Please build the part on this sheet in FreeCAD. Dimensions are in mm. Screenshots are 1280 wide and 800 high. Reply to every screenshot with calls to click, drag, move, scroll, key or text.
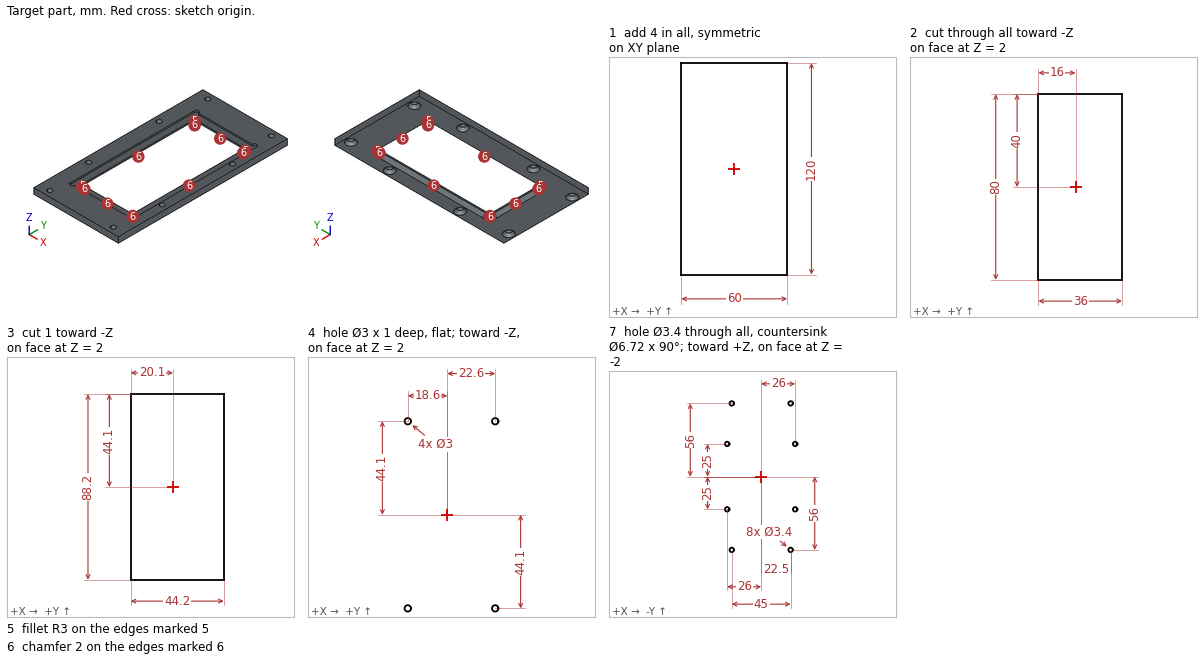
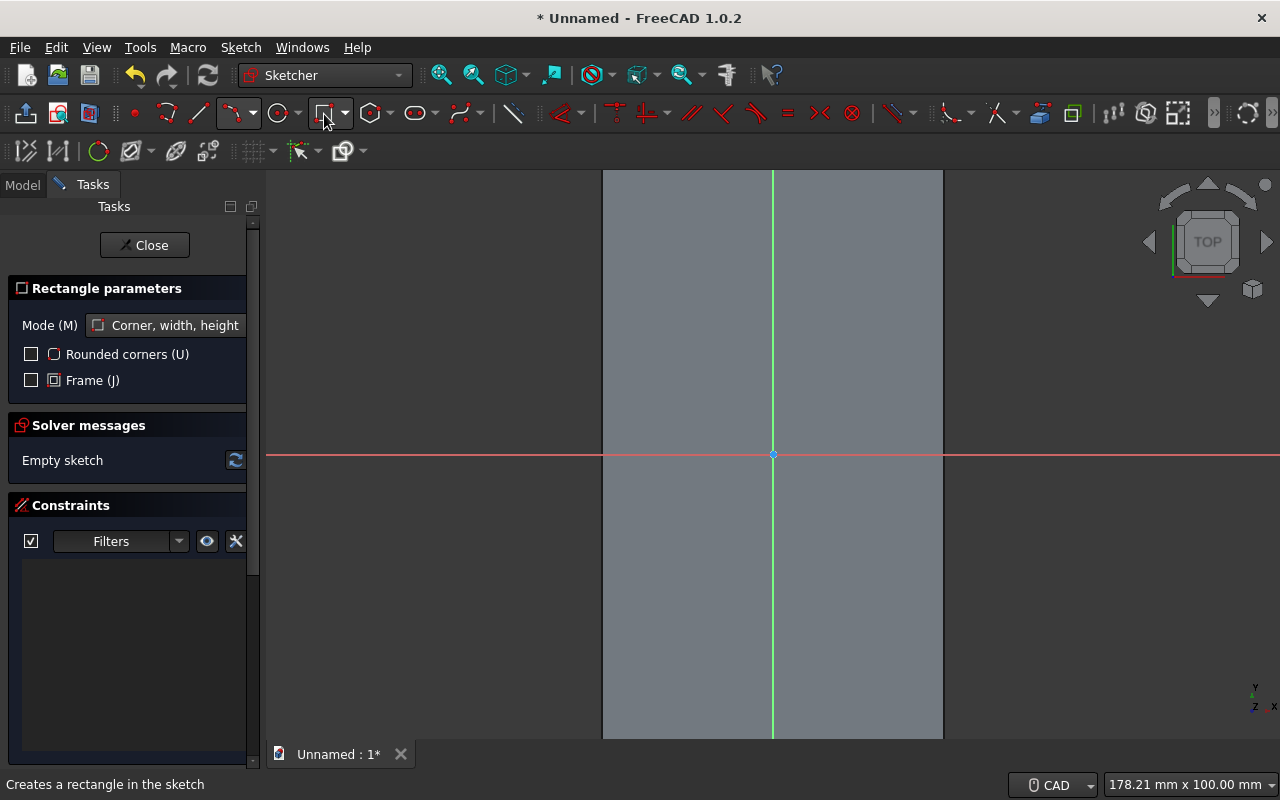
click(682, 227)
click(887, 682)
key(Escape)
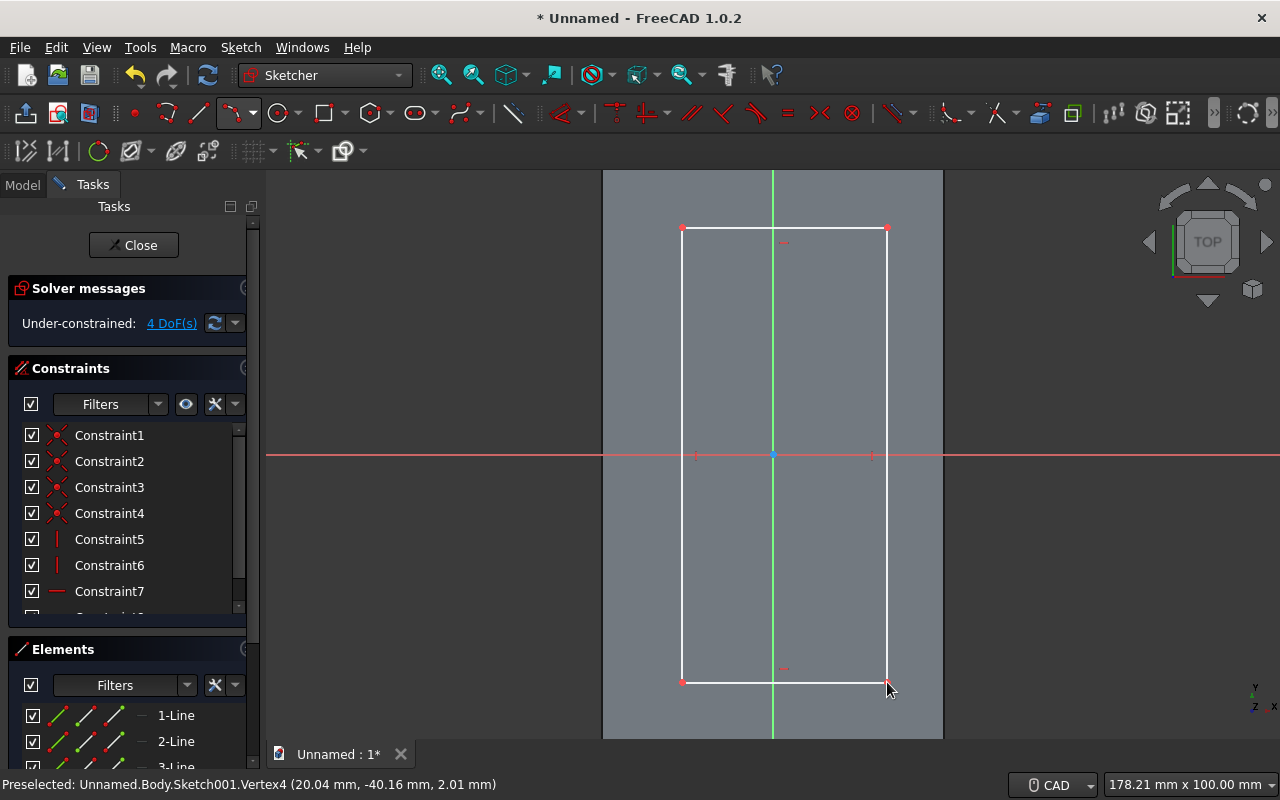
click(560, 114)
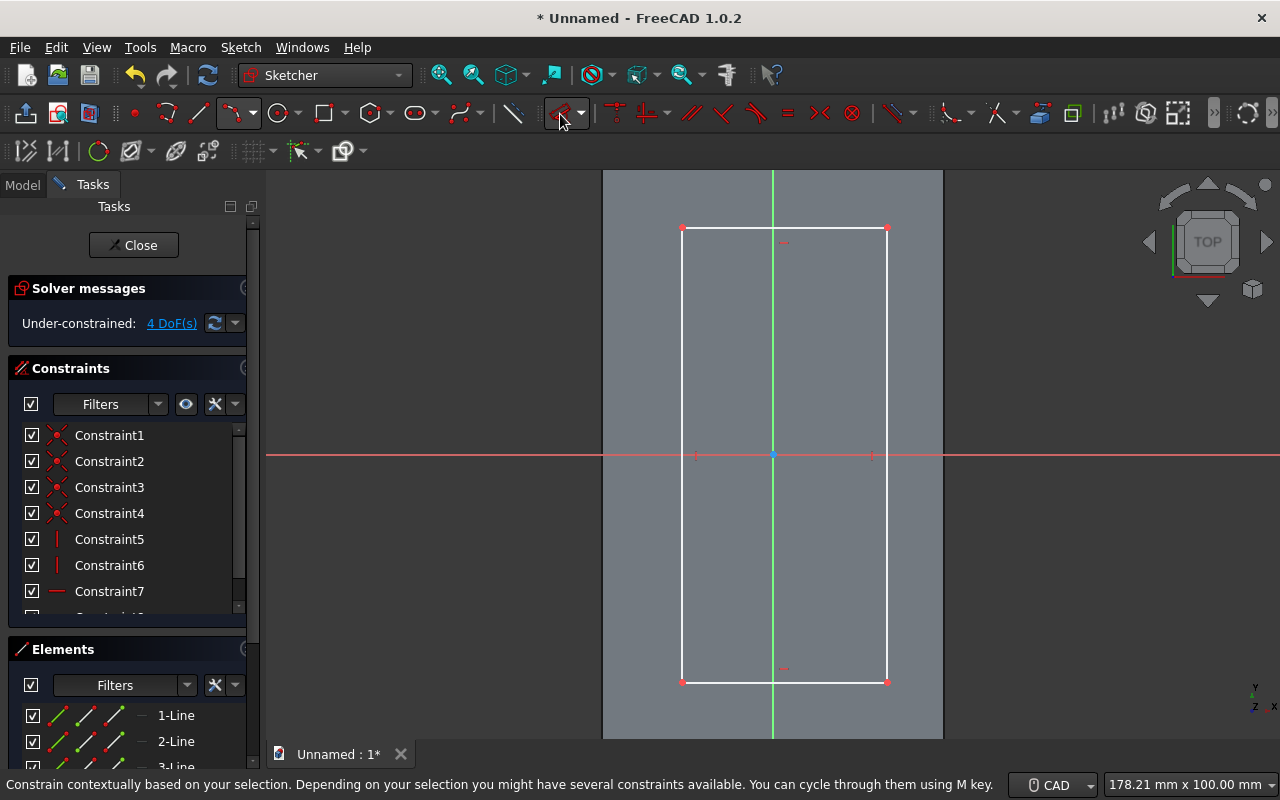
click(682, 365)
click(648, 351)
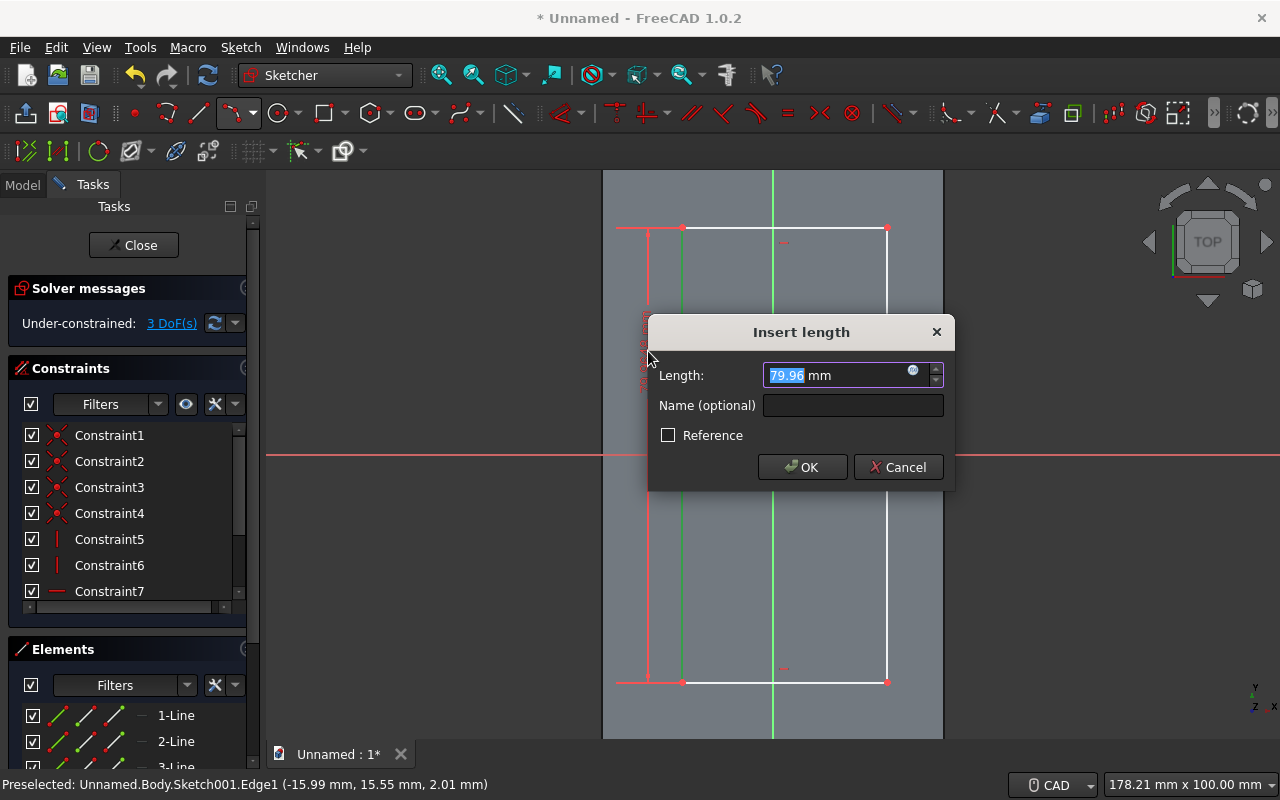
text(80)
key(Return)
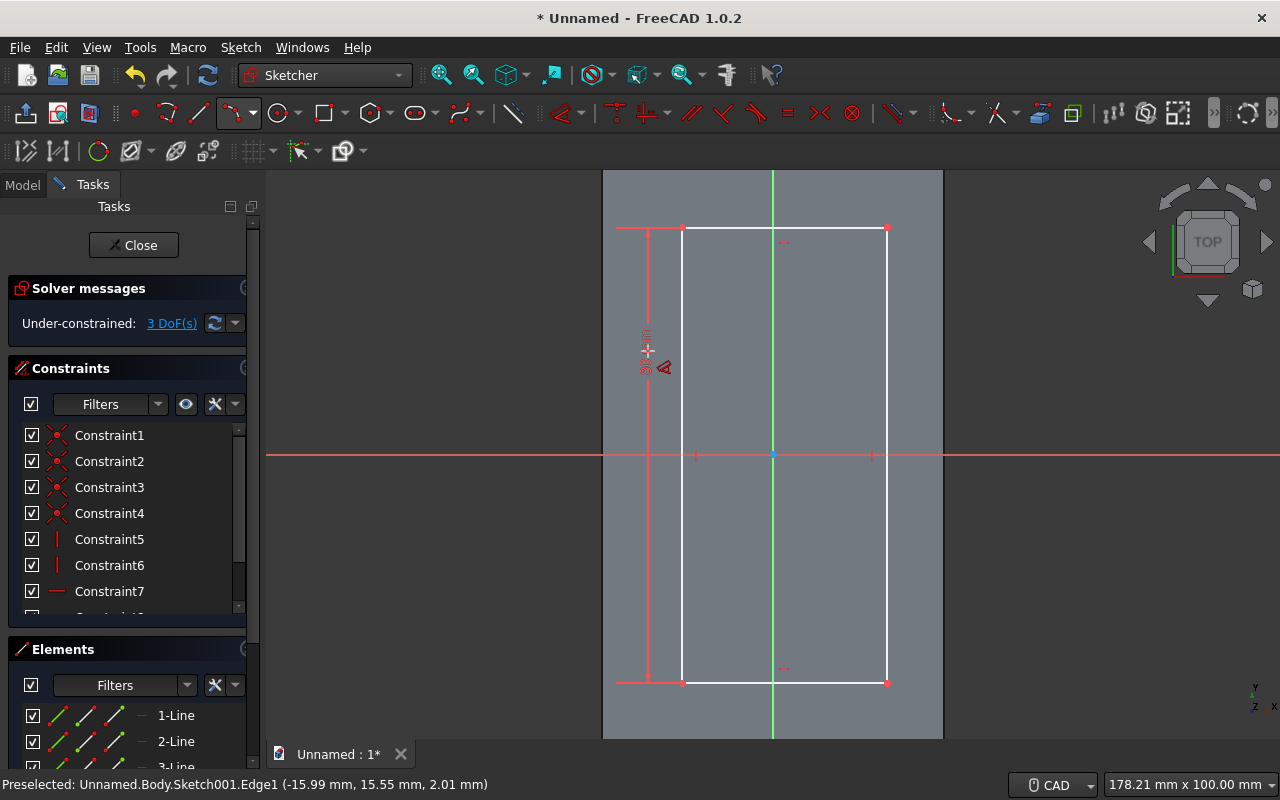
click(743, 683)
click(737, 649)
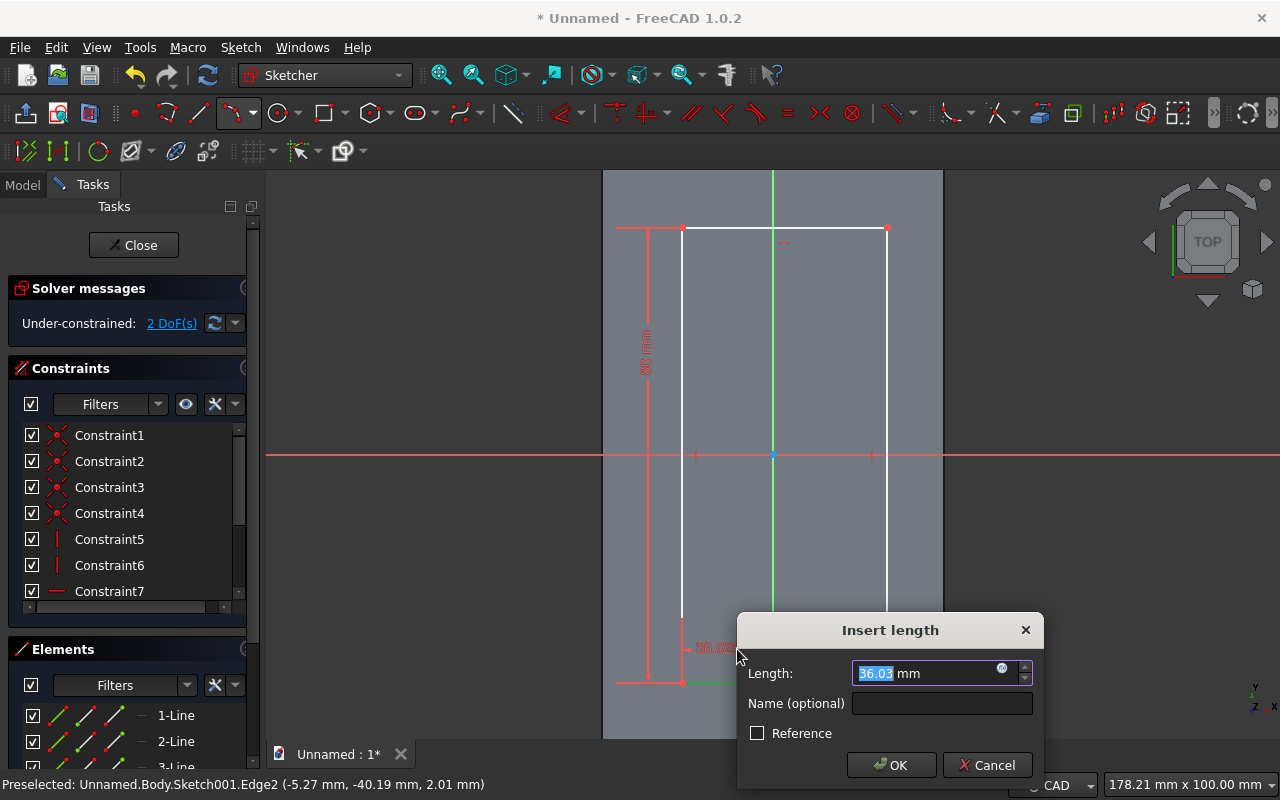
text(36)
key(Return)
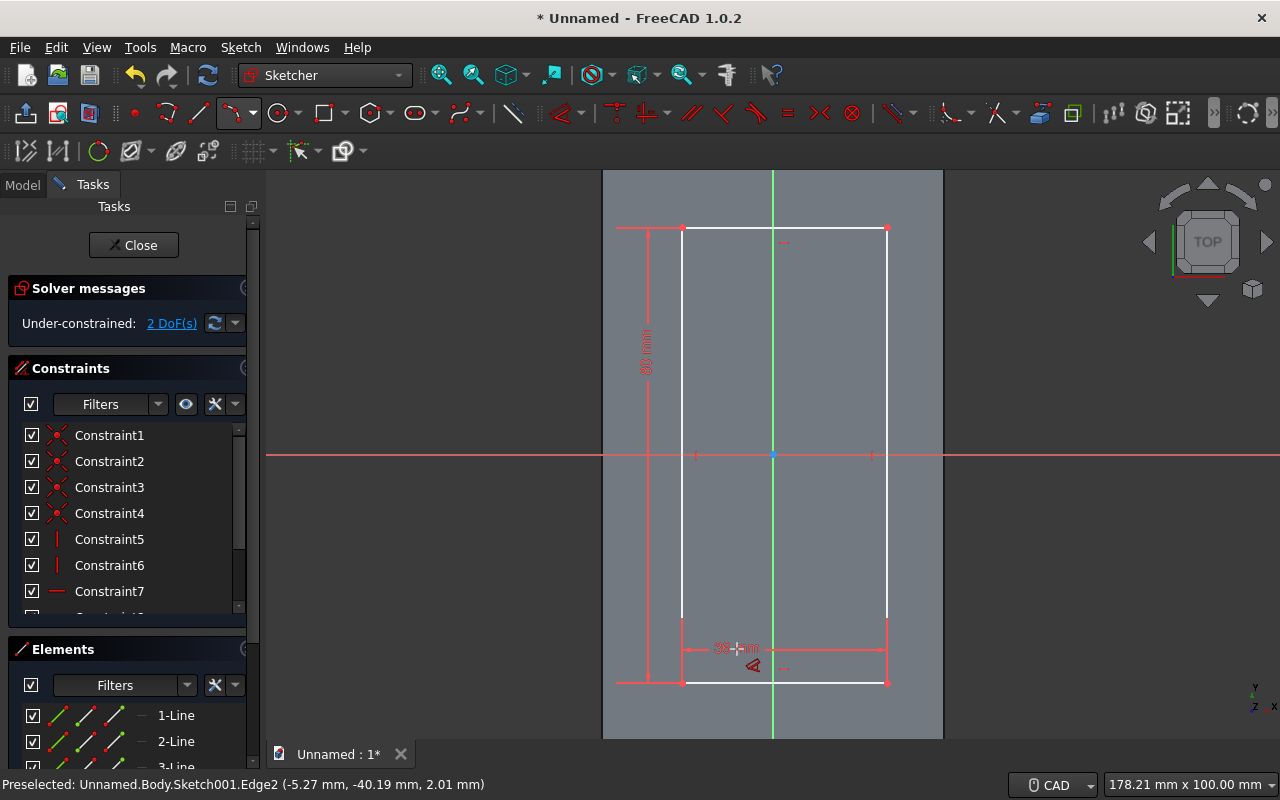
click(682, 228)
click(728, 488)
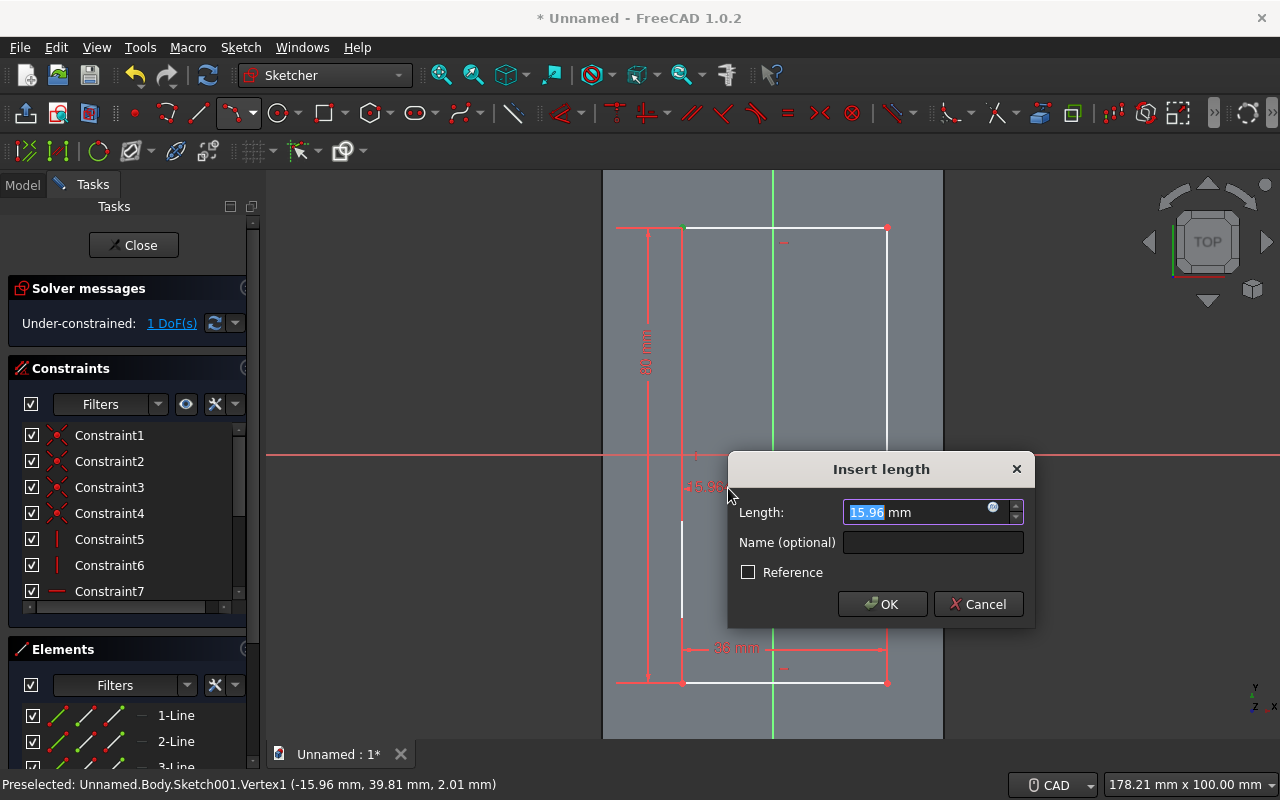
text(16)
key(Return)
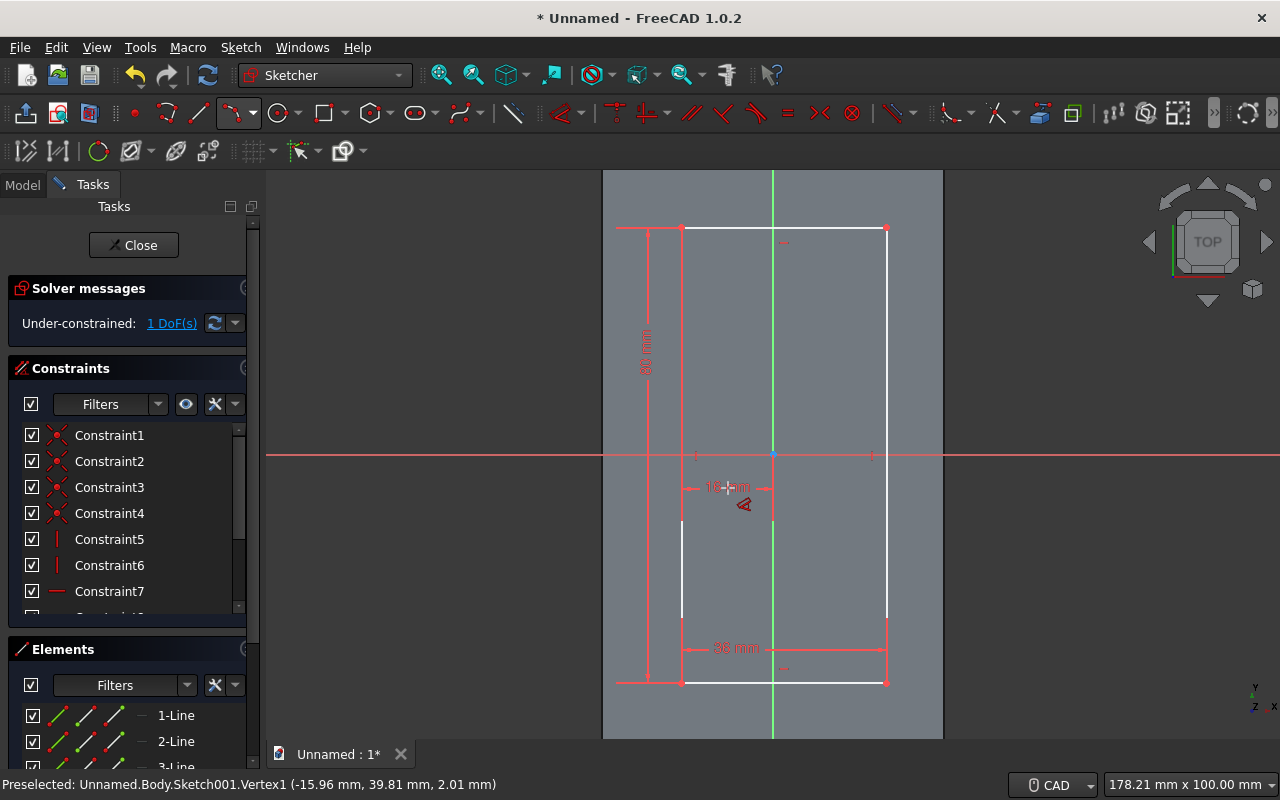
click(682, 228)
click(648, 289)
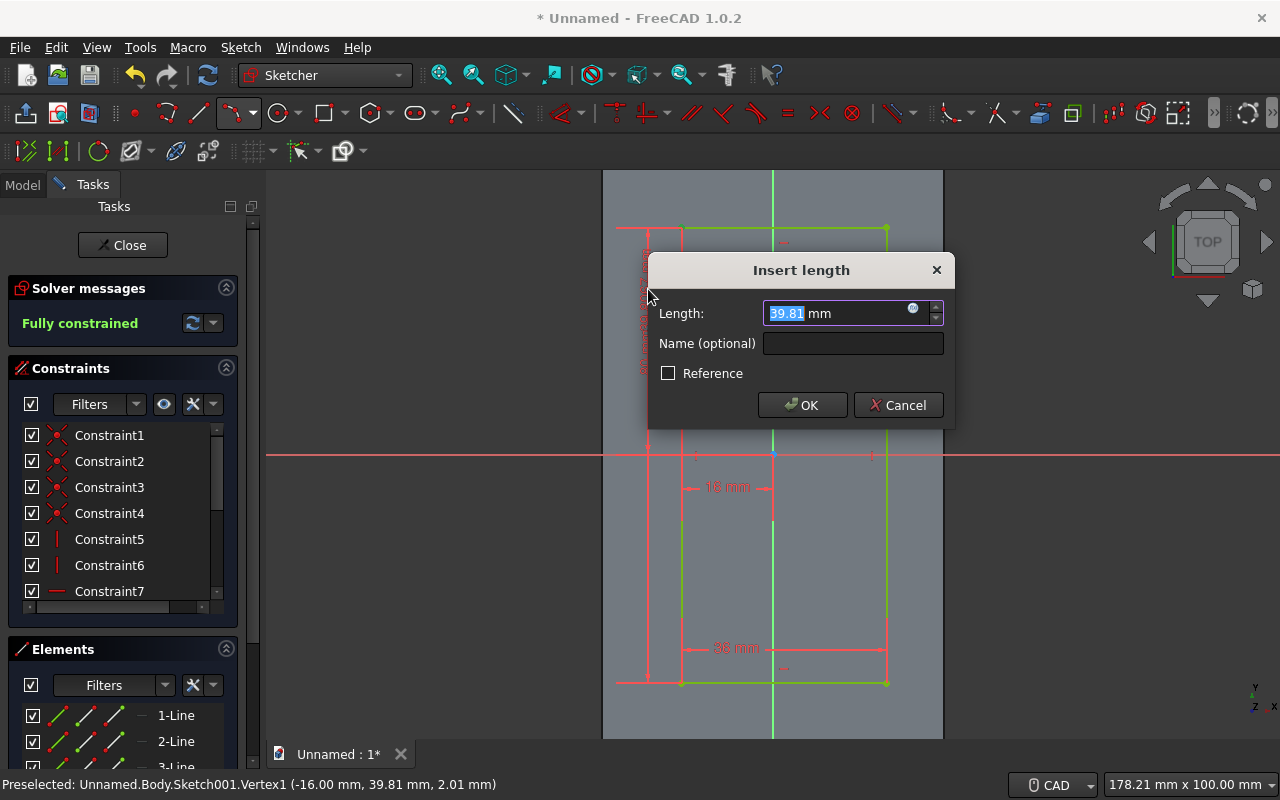
text(40)
key(Return)
key(Escape)